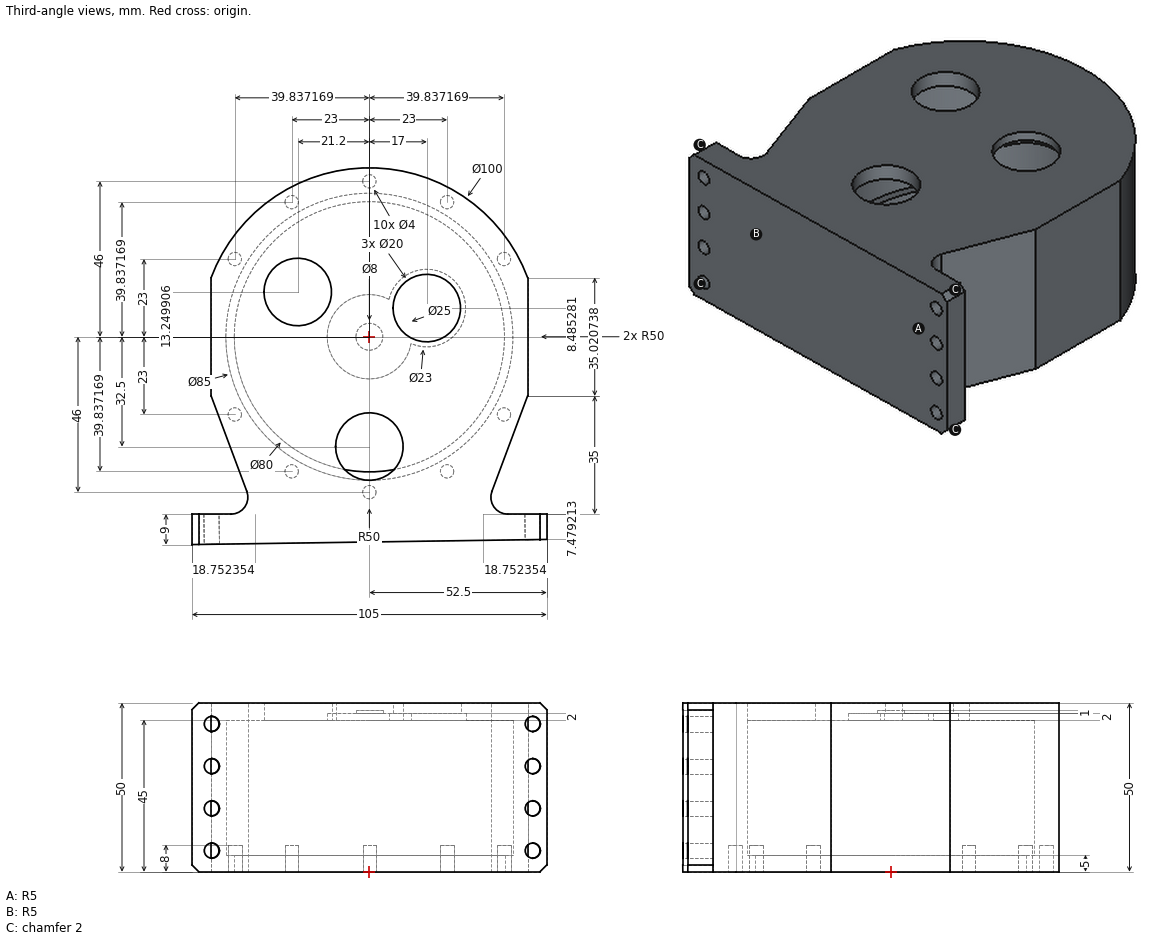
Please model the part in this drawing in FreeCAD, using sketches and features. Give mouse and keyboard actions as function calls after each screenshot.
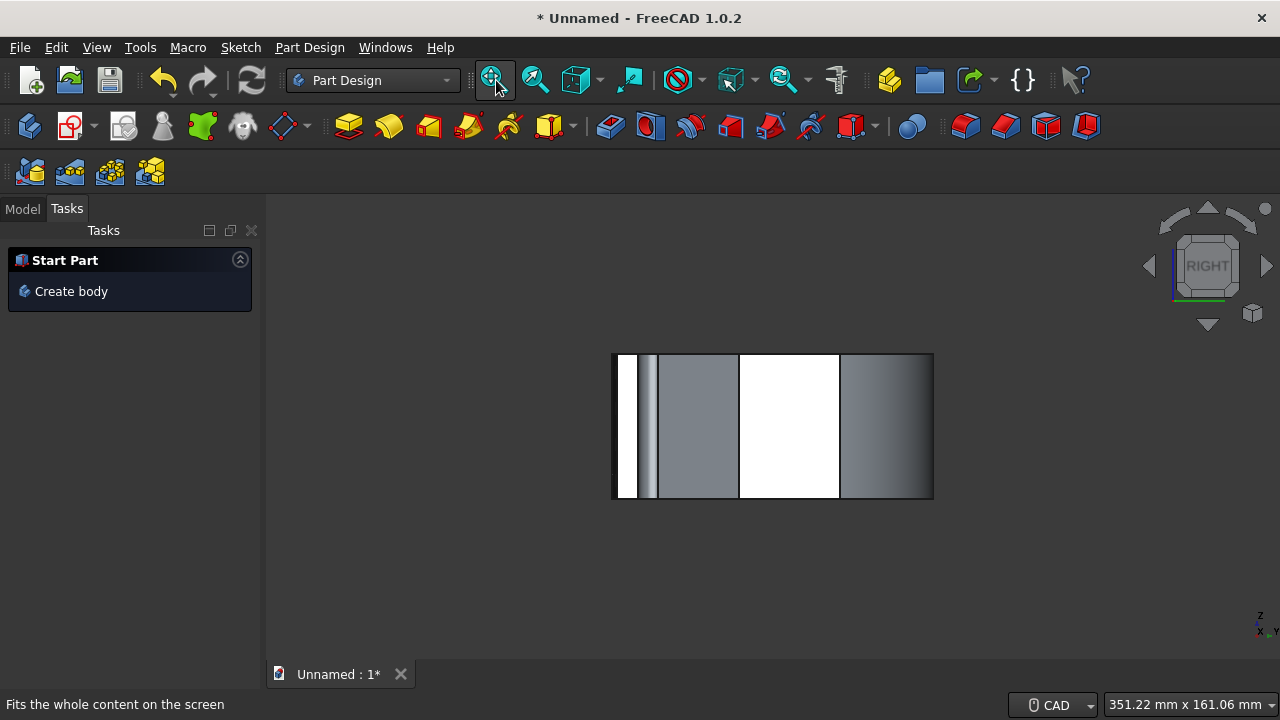
key(5)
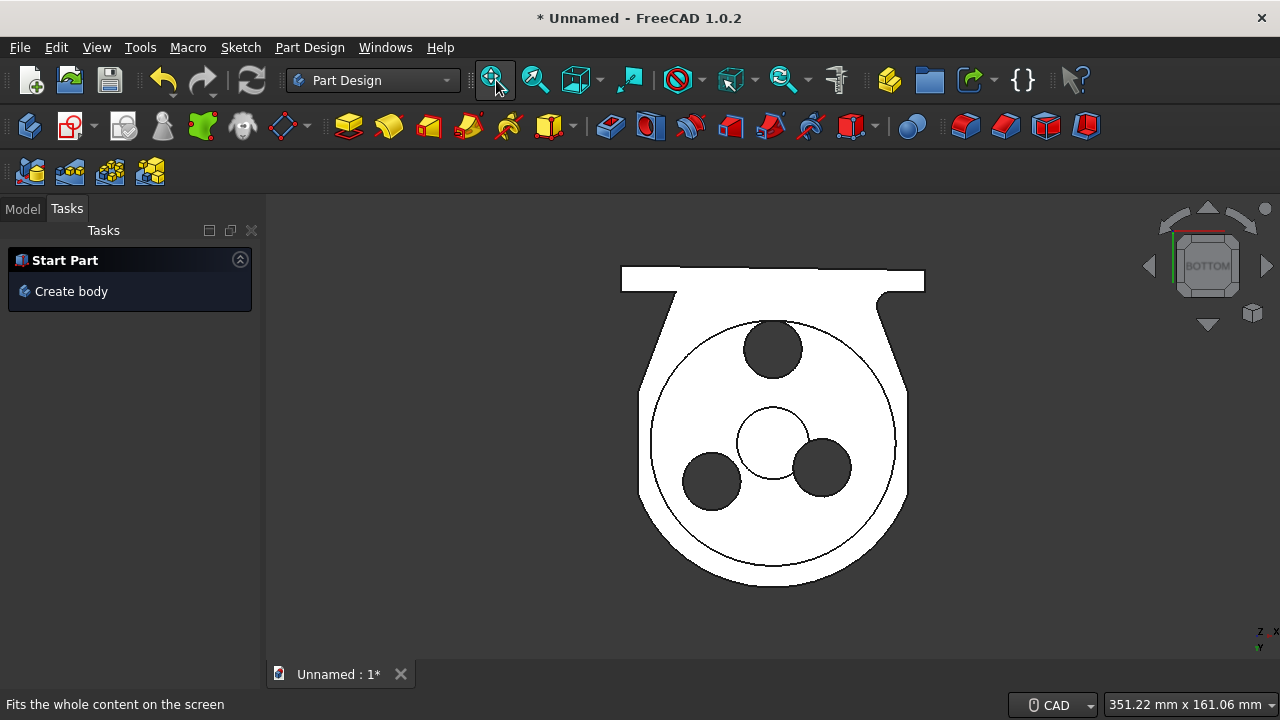
key(4)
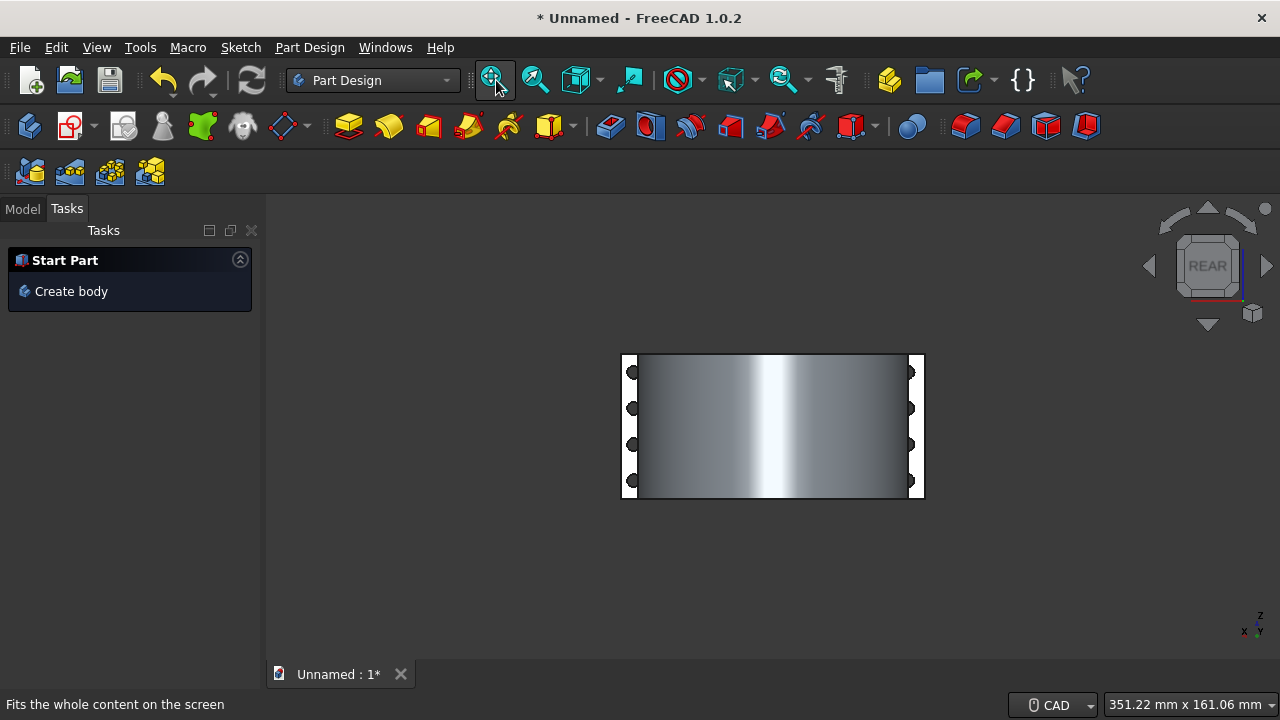
click(496, 80)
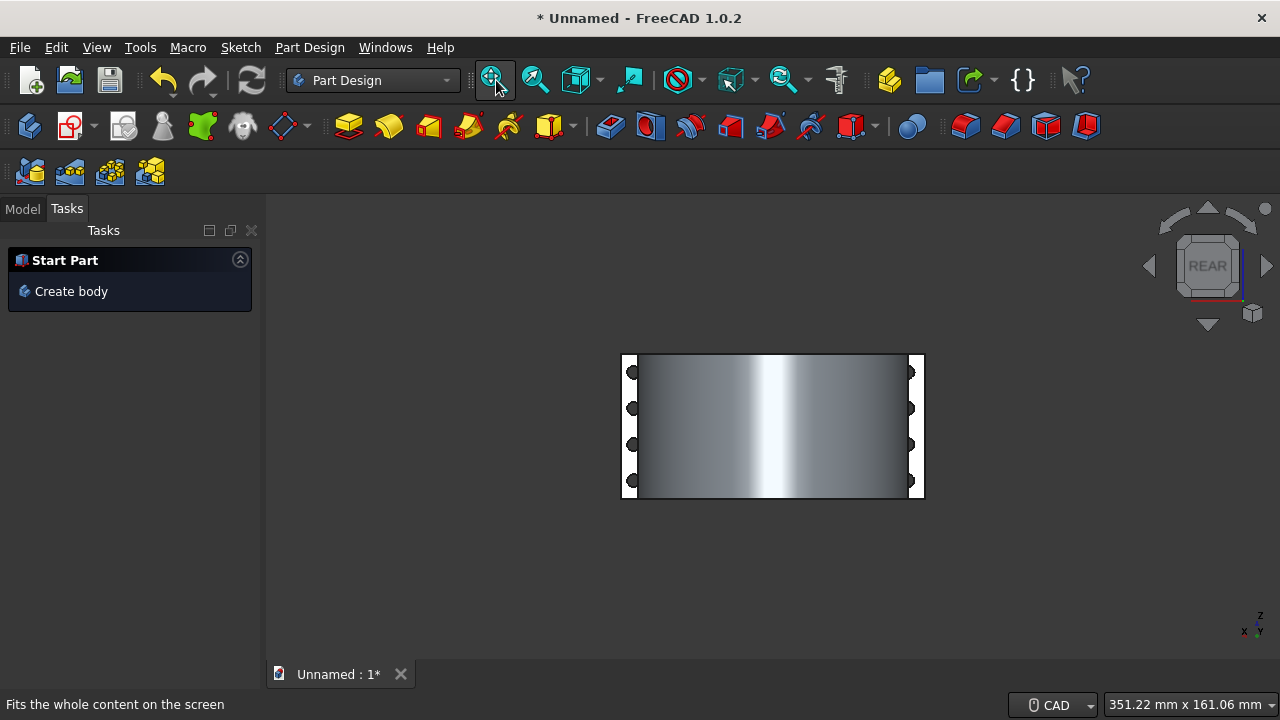
key(6)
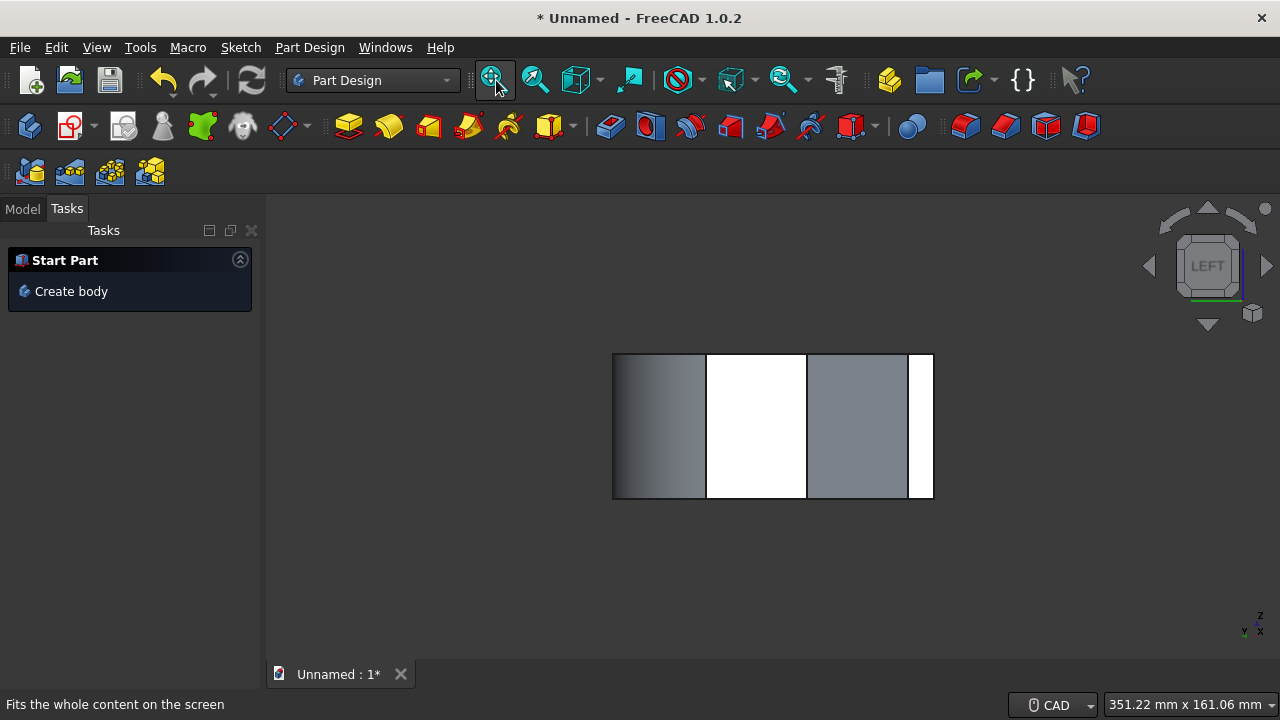
click(496, 80)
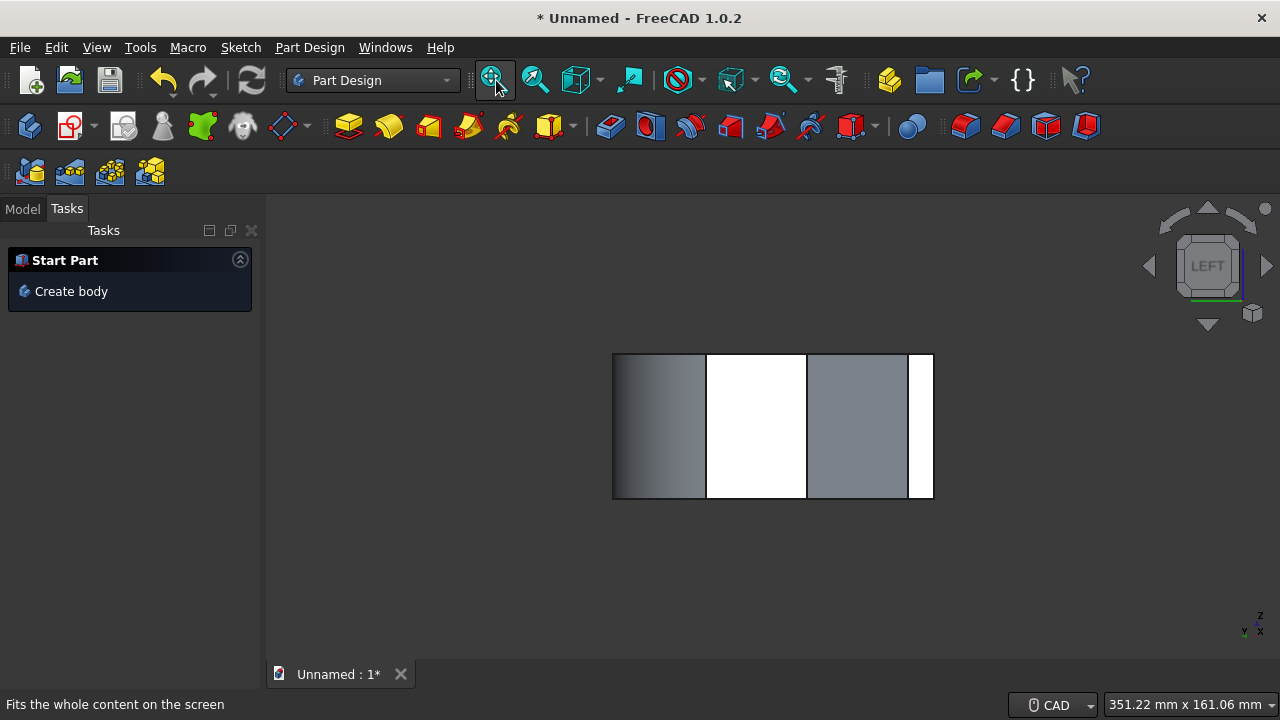
key(v)
key(3)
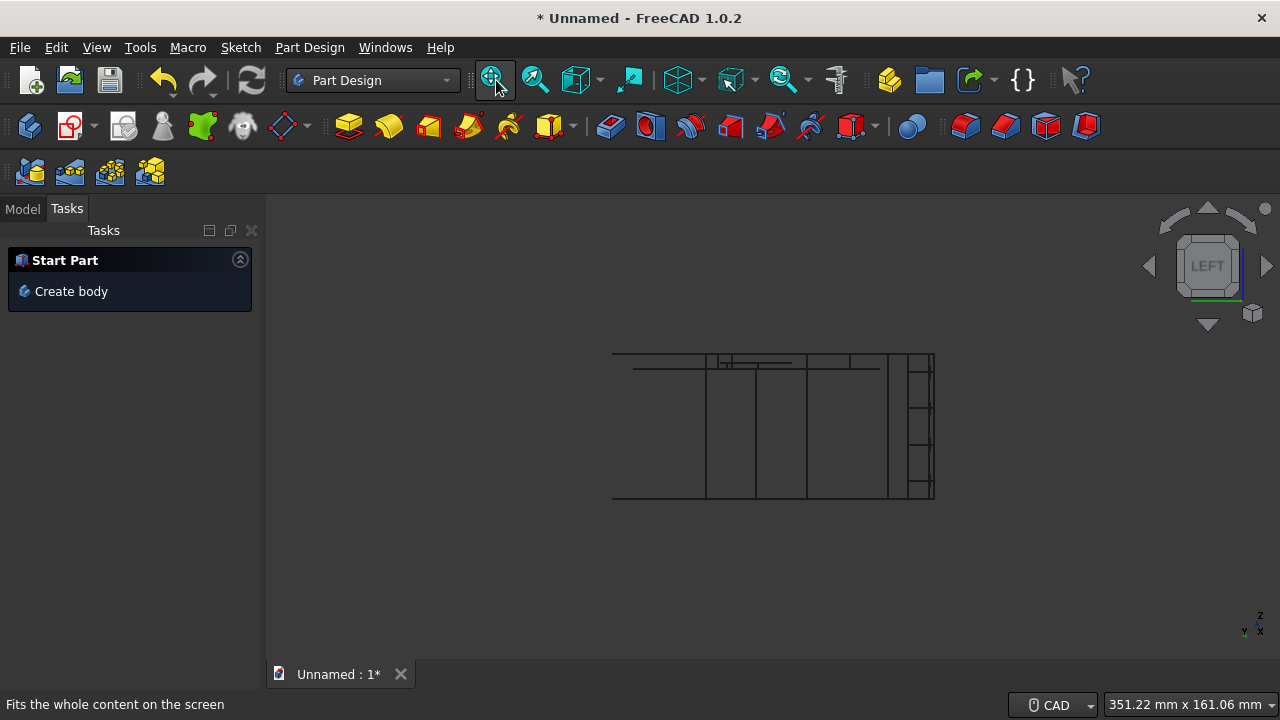
key(0)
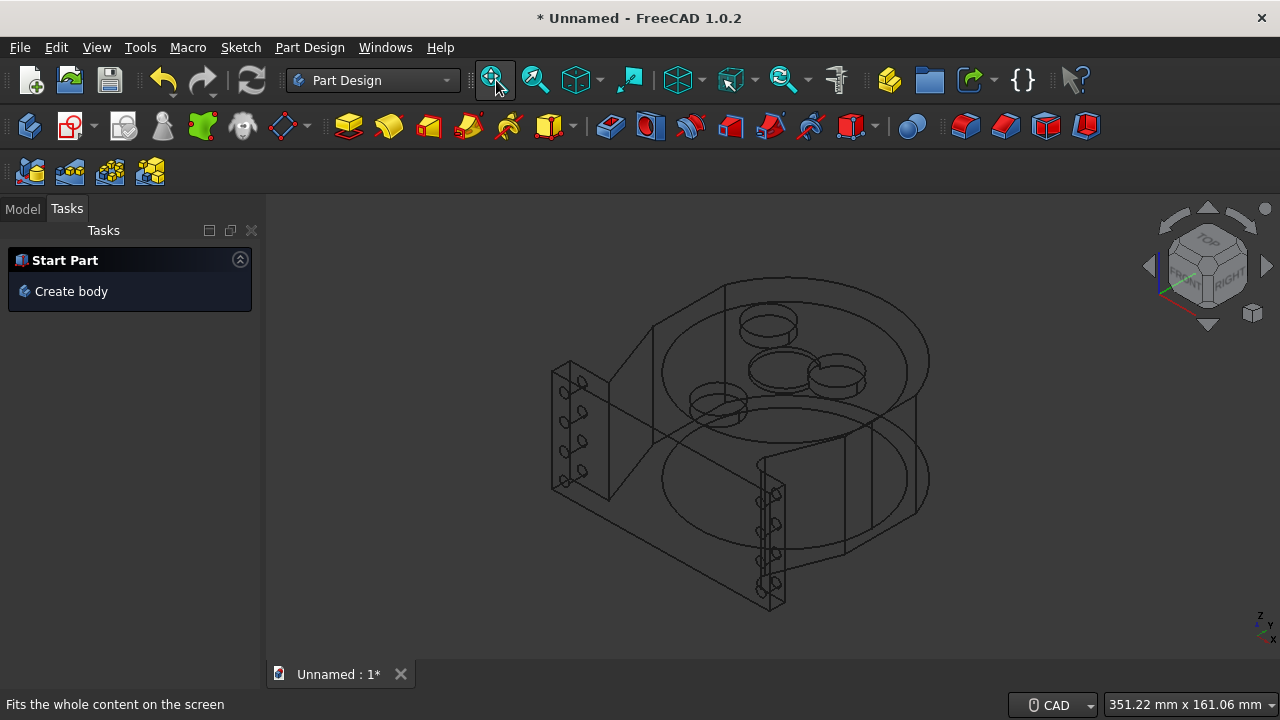
click(609, 441)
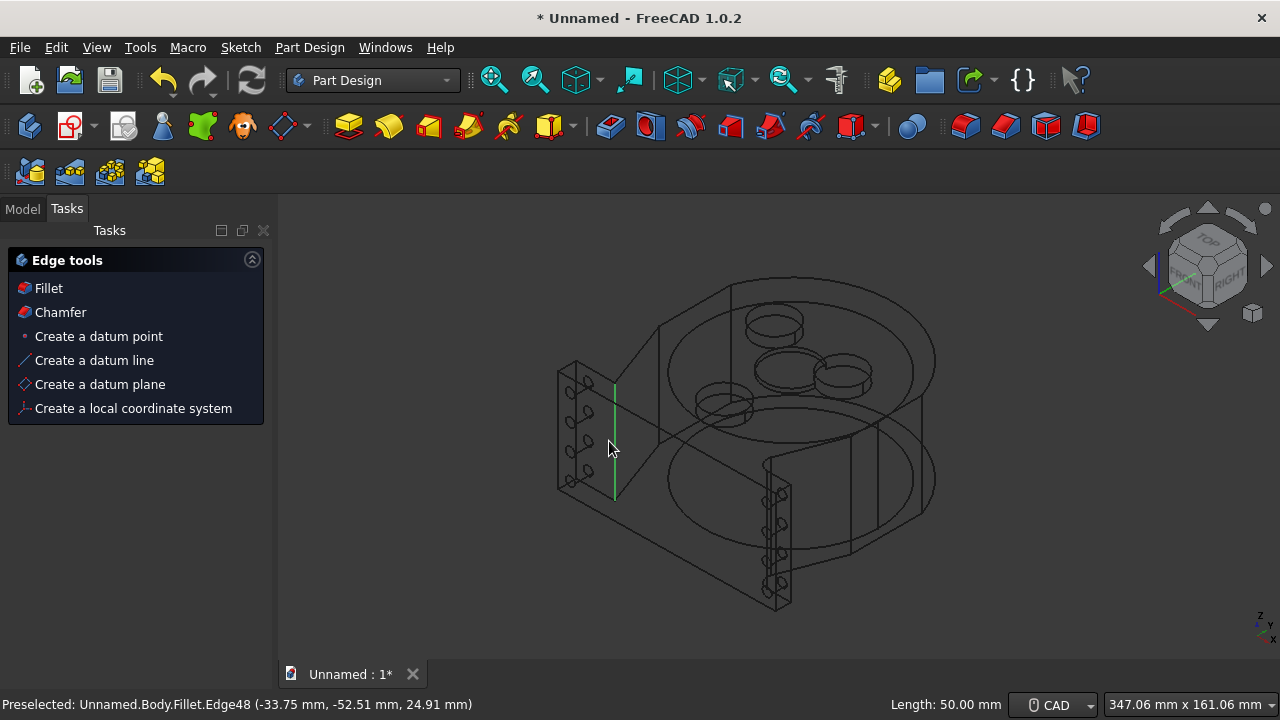
key(v)
key(1)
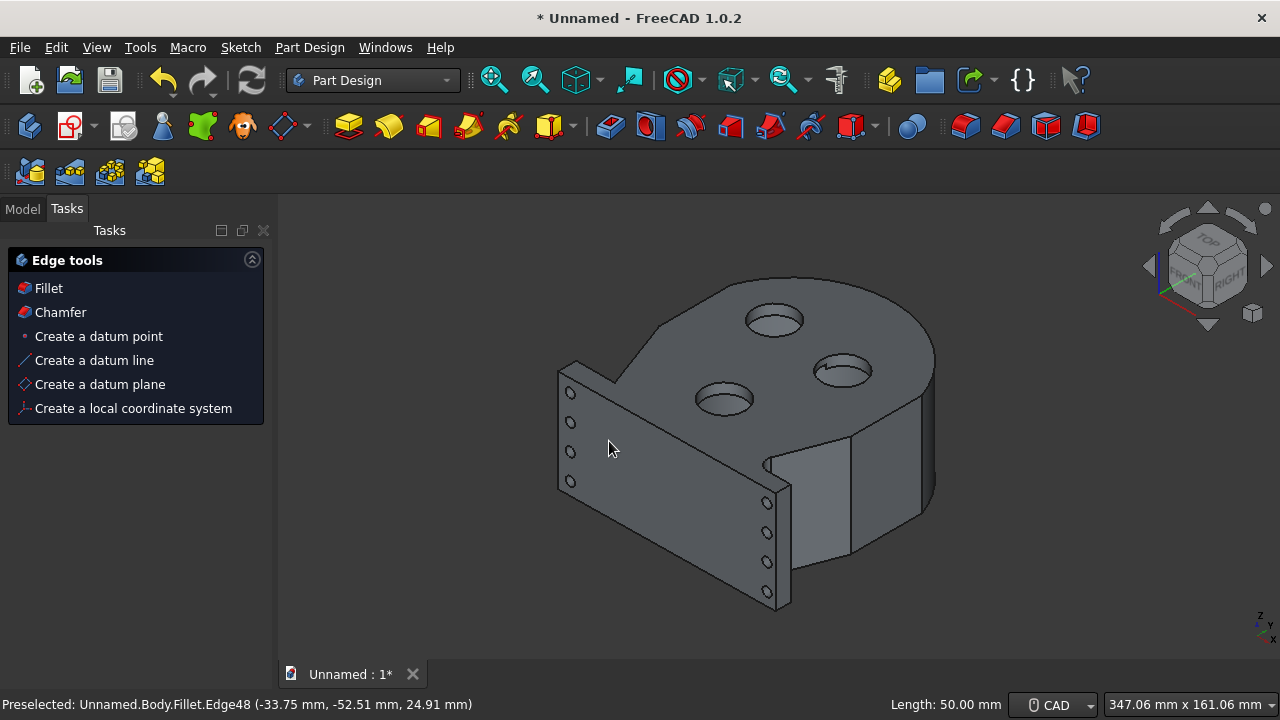
click(966, 126)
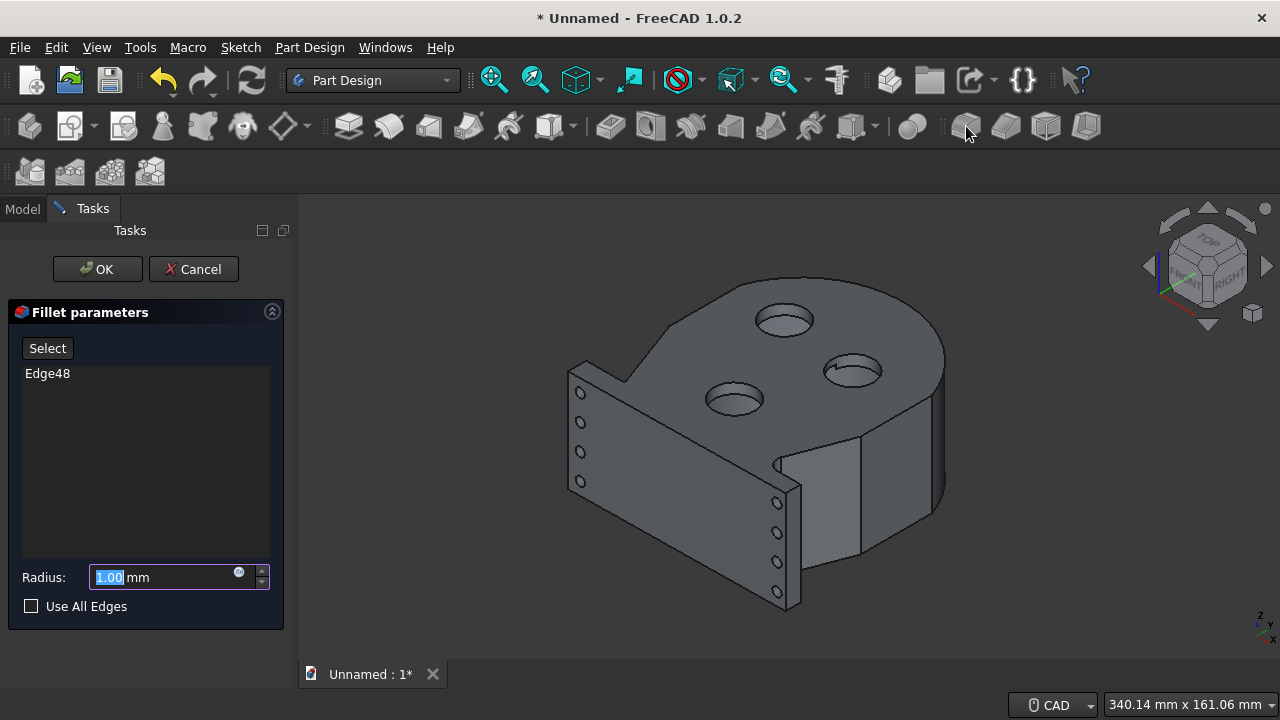
text(5)
key(Tab)